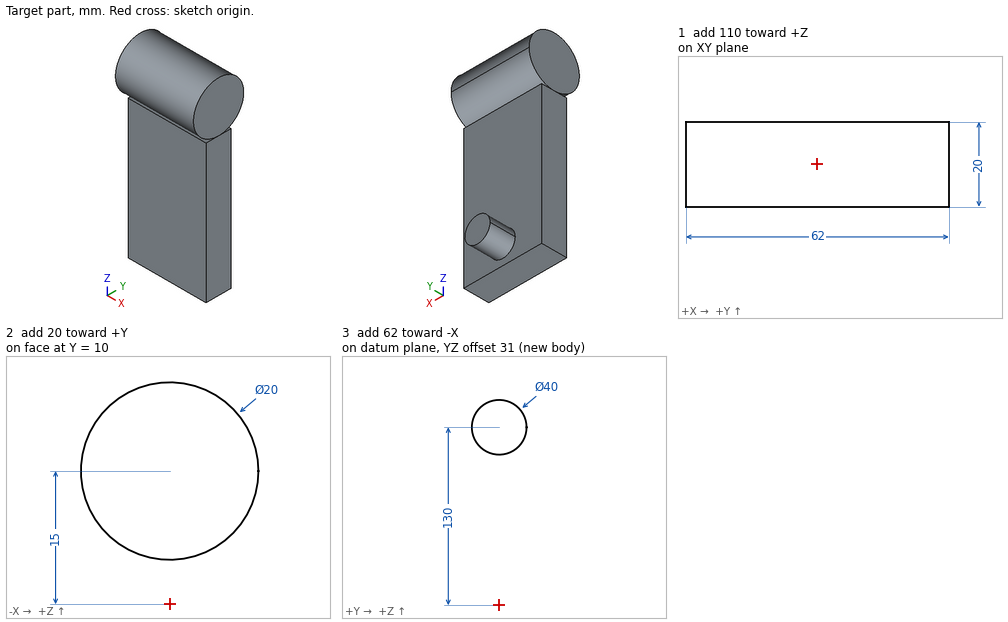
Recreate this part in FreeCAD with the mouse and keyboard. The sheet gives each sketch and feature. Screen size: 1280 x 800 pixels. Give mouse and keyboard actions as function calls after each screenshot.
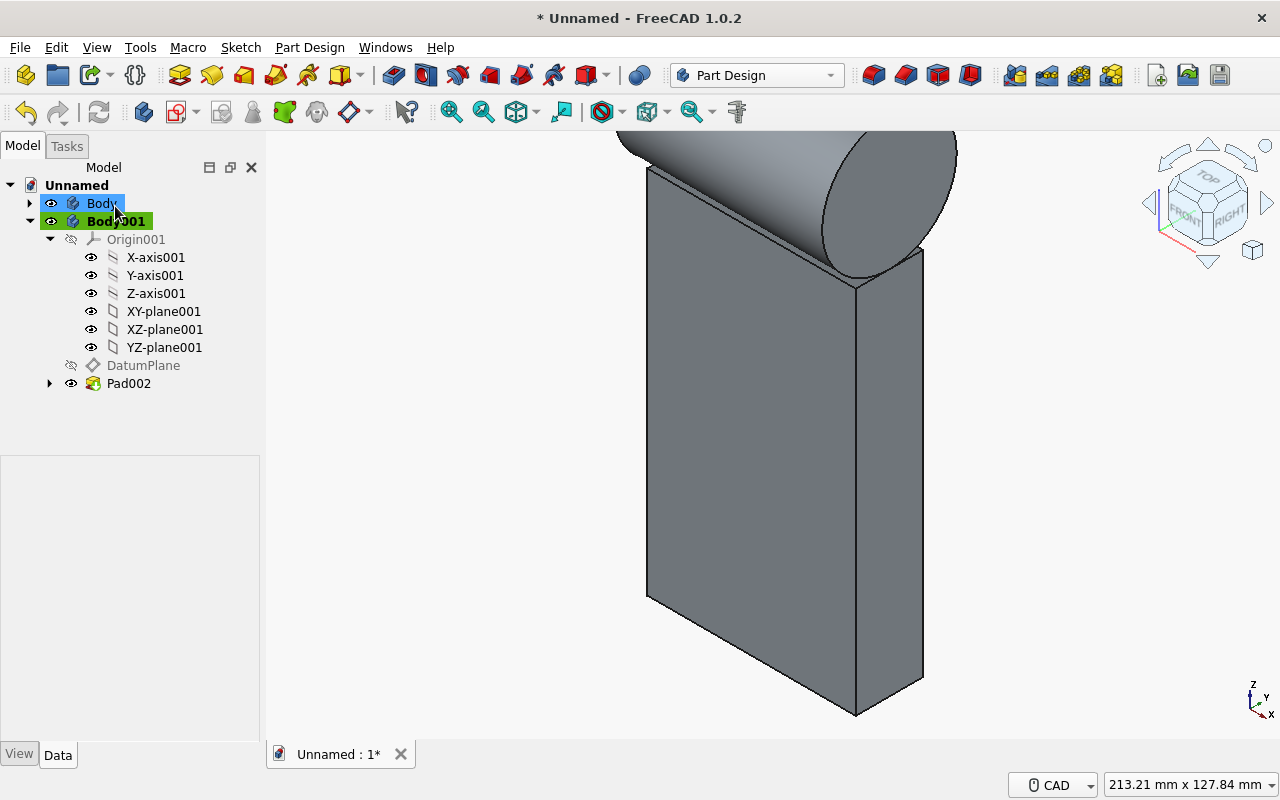
key(v)
key(f)